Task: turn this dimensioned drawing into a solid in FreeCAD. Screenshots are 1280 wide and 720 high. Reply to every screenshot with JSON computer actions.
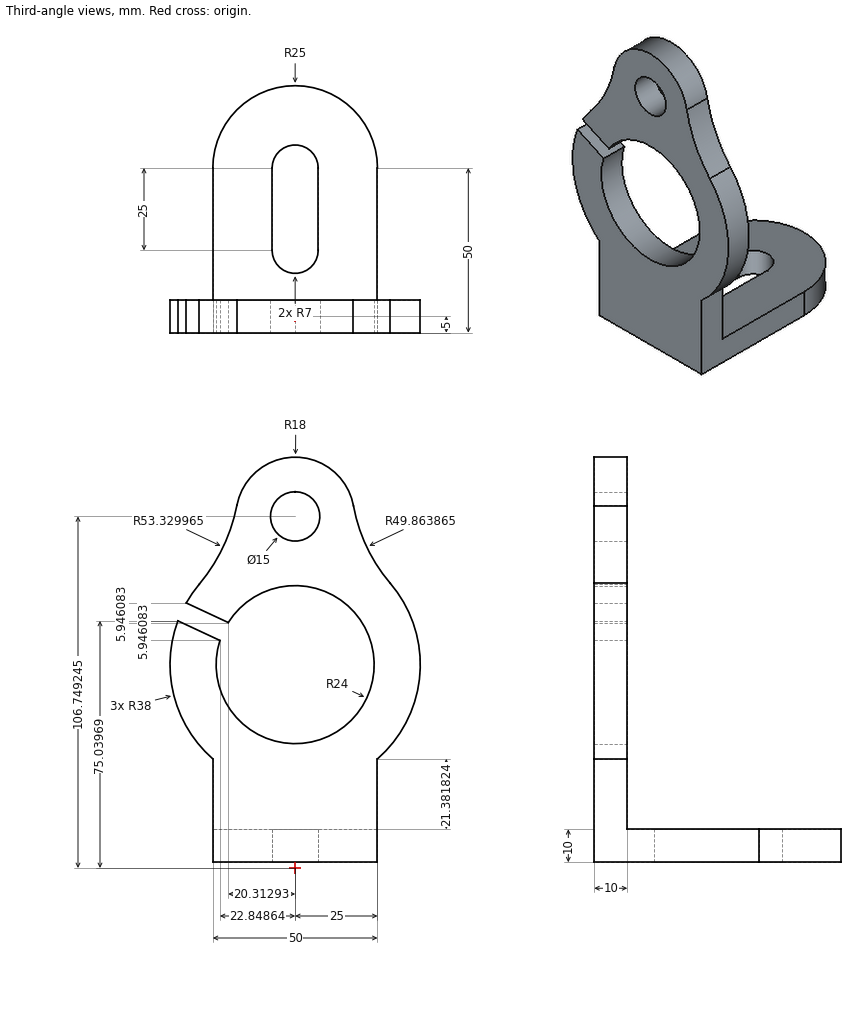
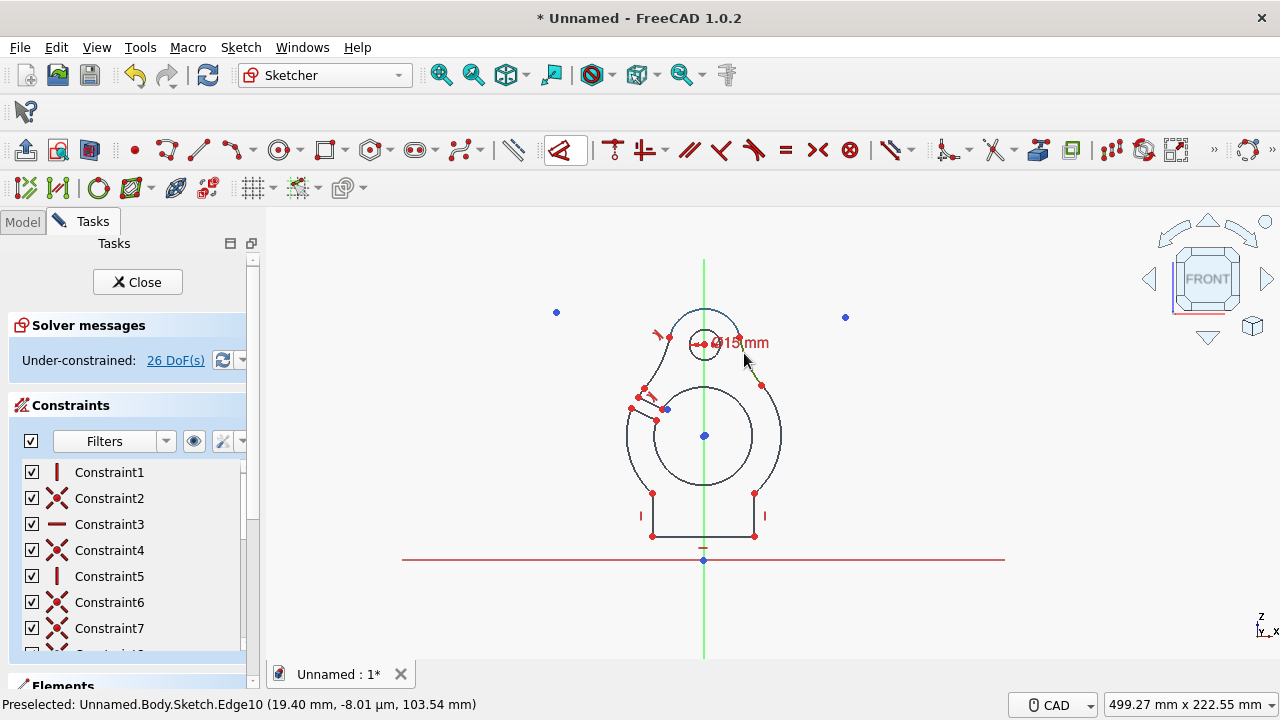
{"action": "left_click", "coordinate": [754, 150]}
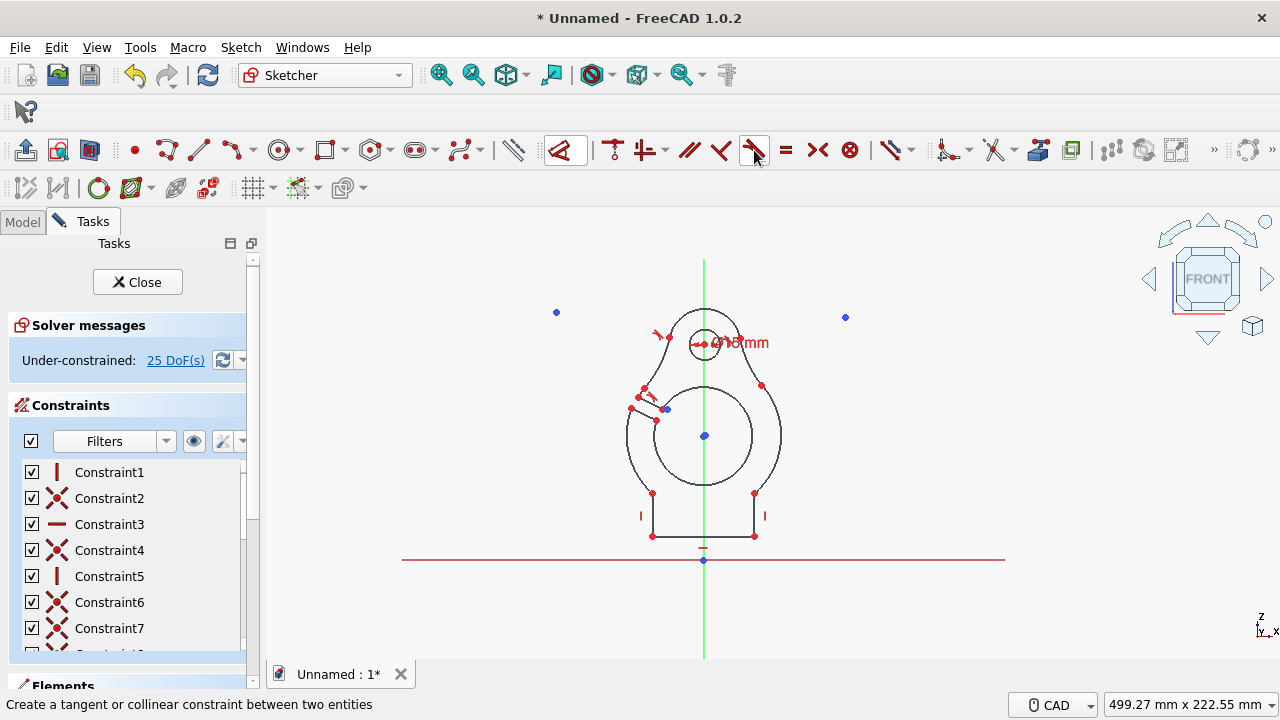
{"action": "left_click", "coordinate": [744, 353]}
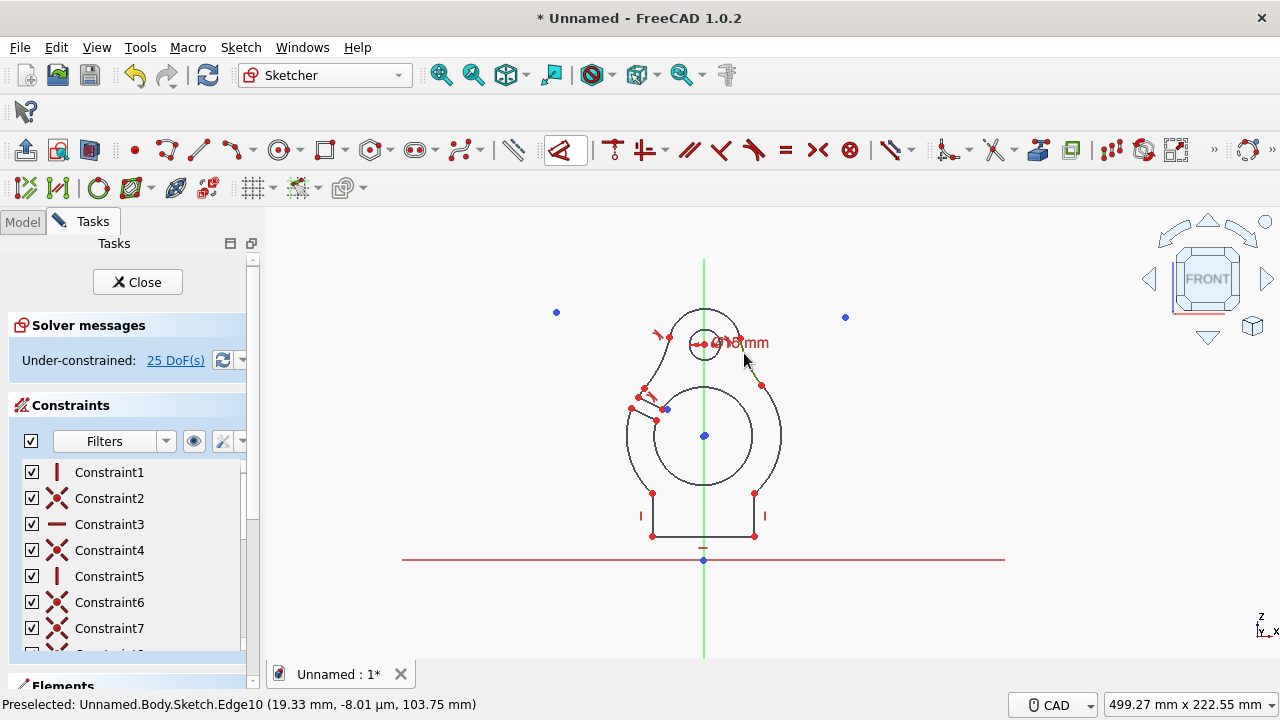
{"action": "left_click", "coordinate": [775, 465]}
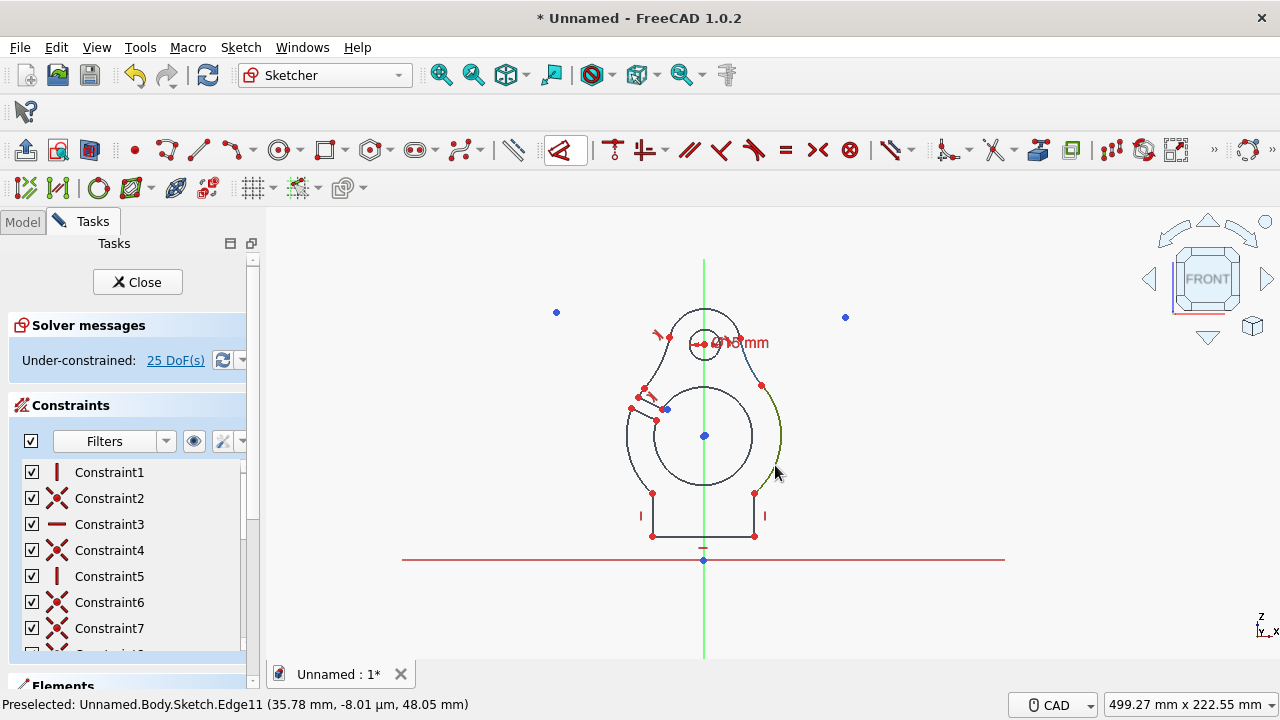
{"action": "key", "text": "t"}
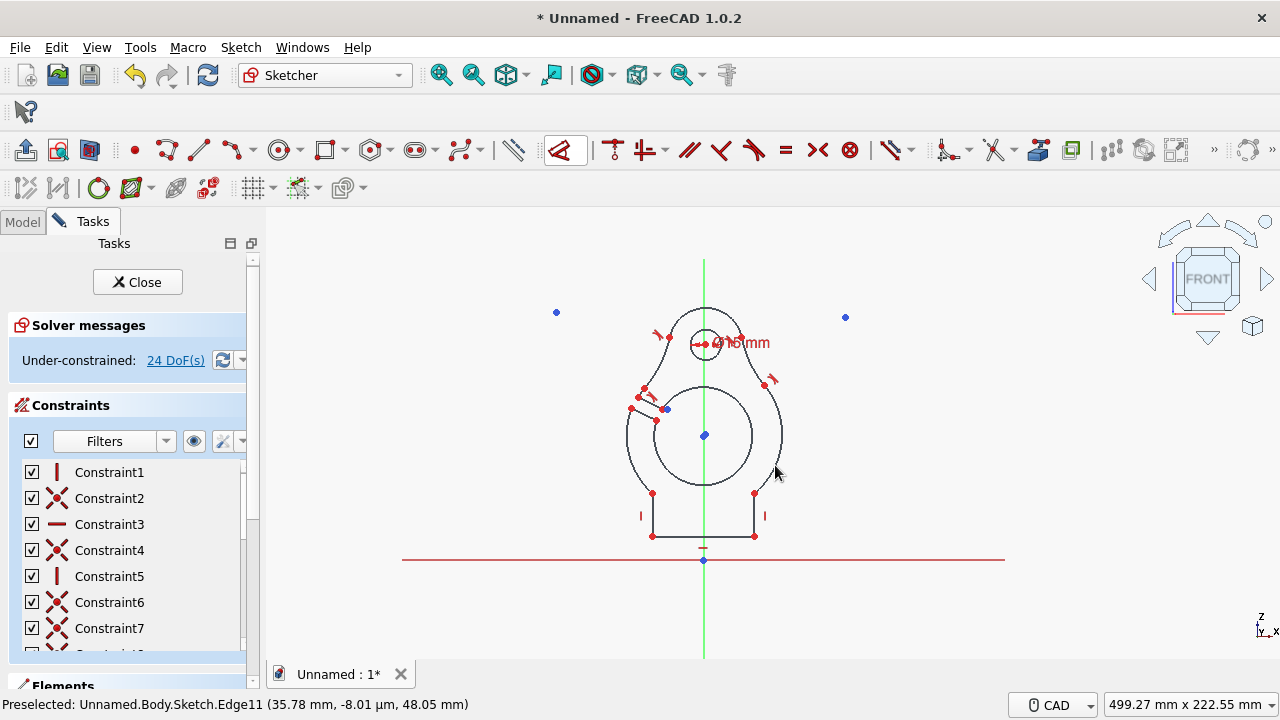
{"action": "left_click", "coordinate": [739, 403]}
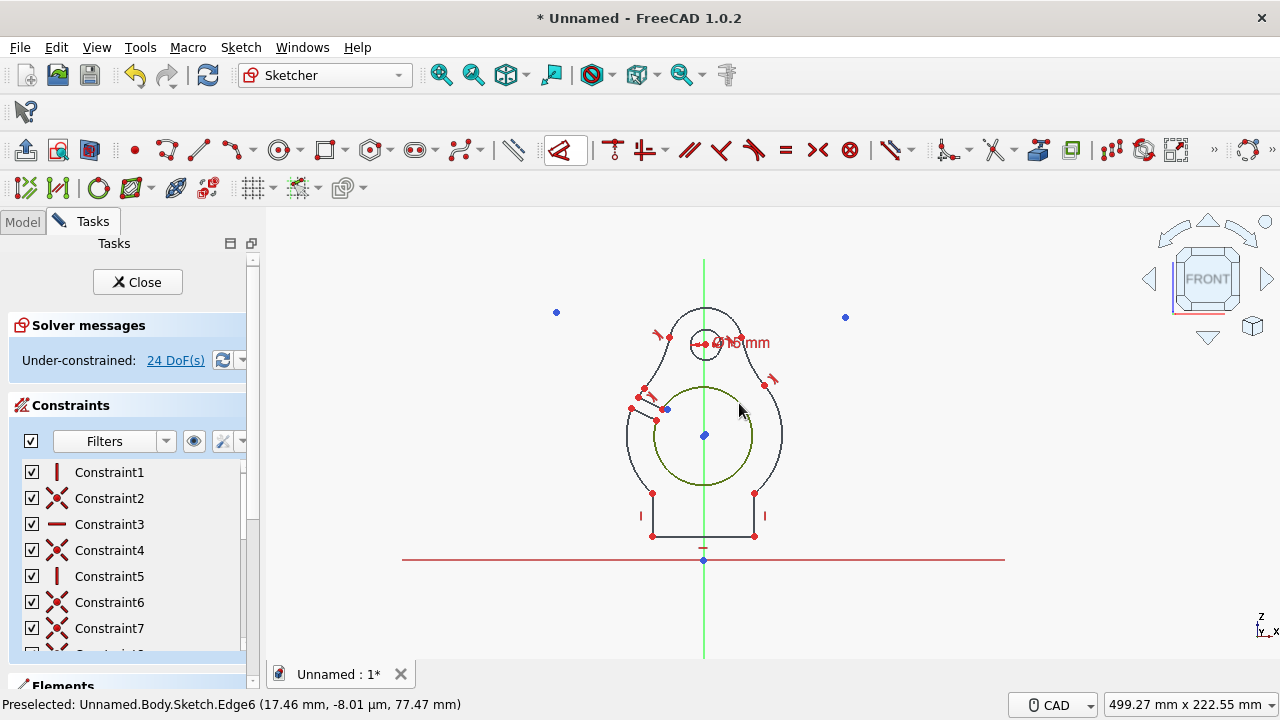
{"action": "scroll", "coordinate": [641, 393], "scroll_direction": "up", "scroll_amount": 6}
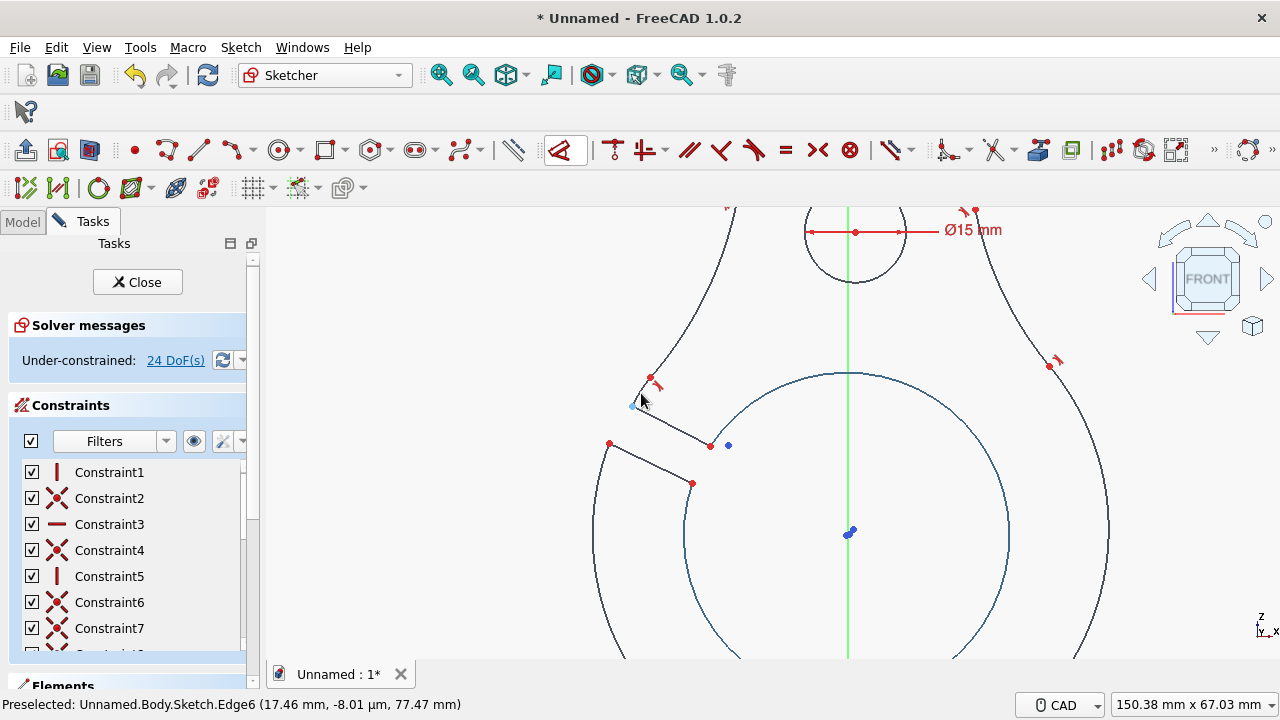
{"action": "left_click", "coordinate": [640, 391]}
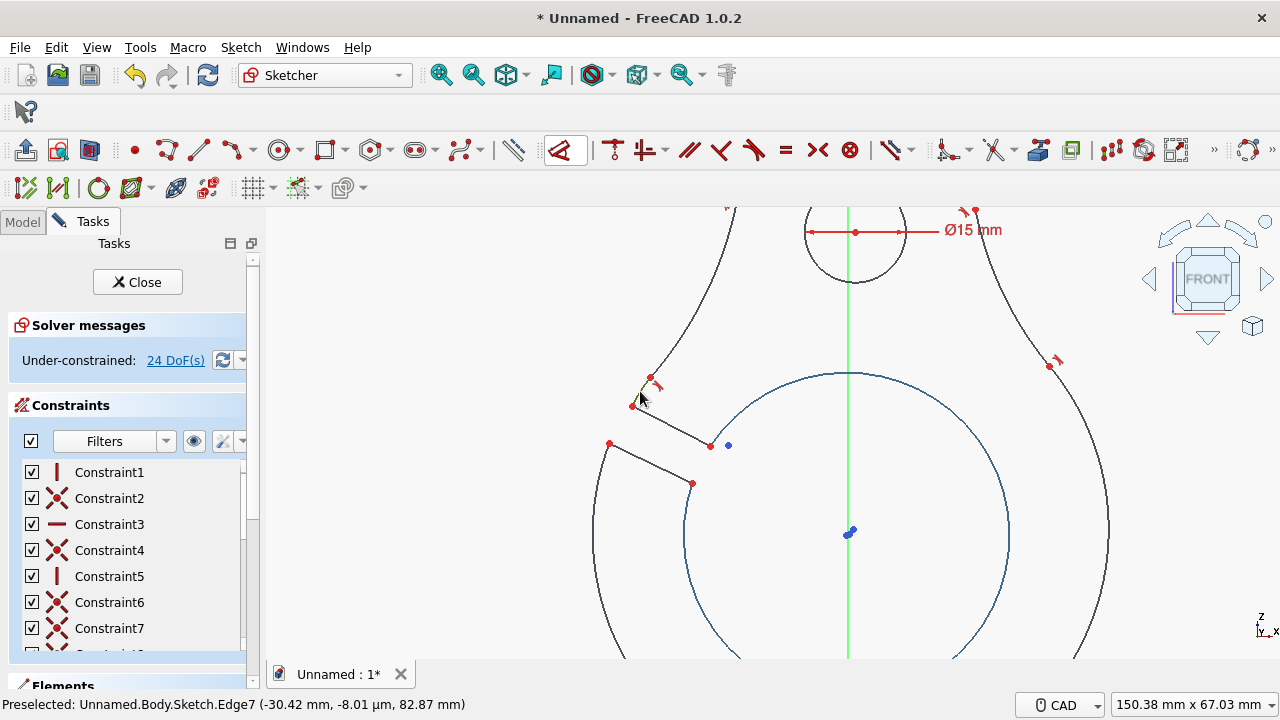
{"action": "left_click", "coordinate": [614, 150]}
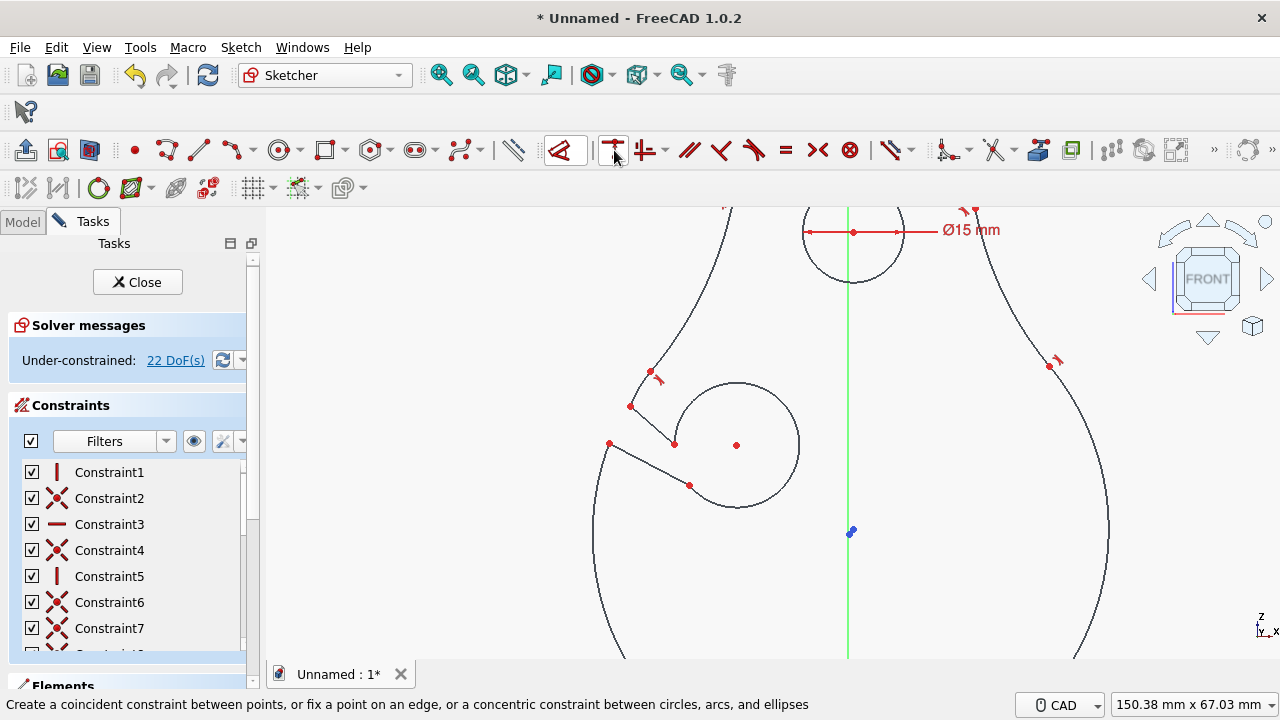
{"action": "left_click", "coordinate": [782, 489]}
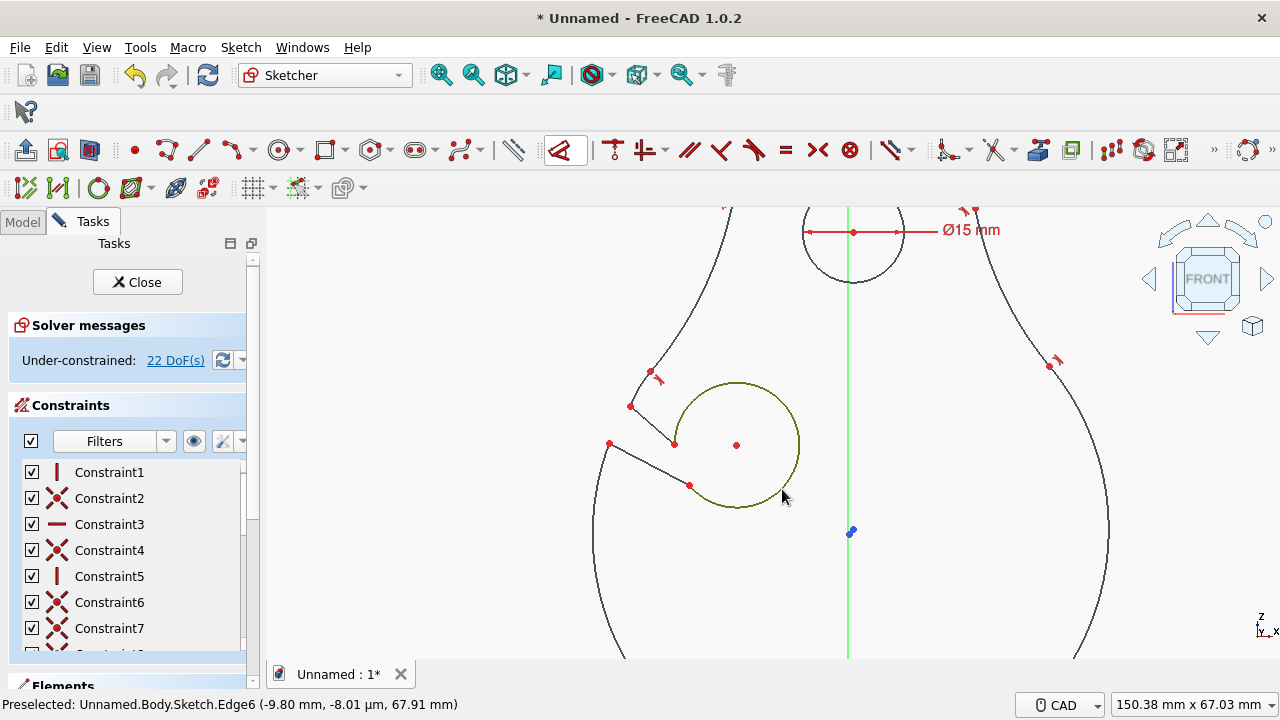
{"action": "left_click", "coordinate": [1103, 474]}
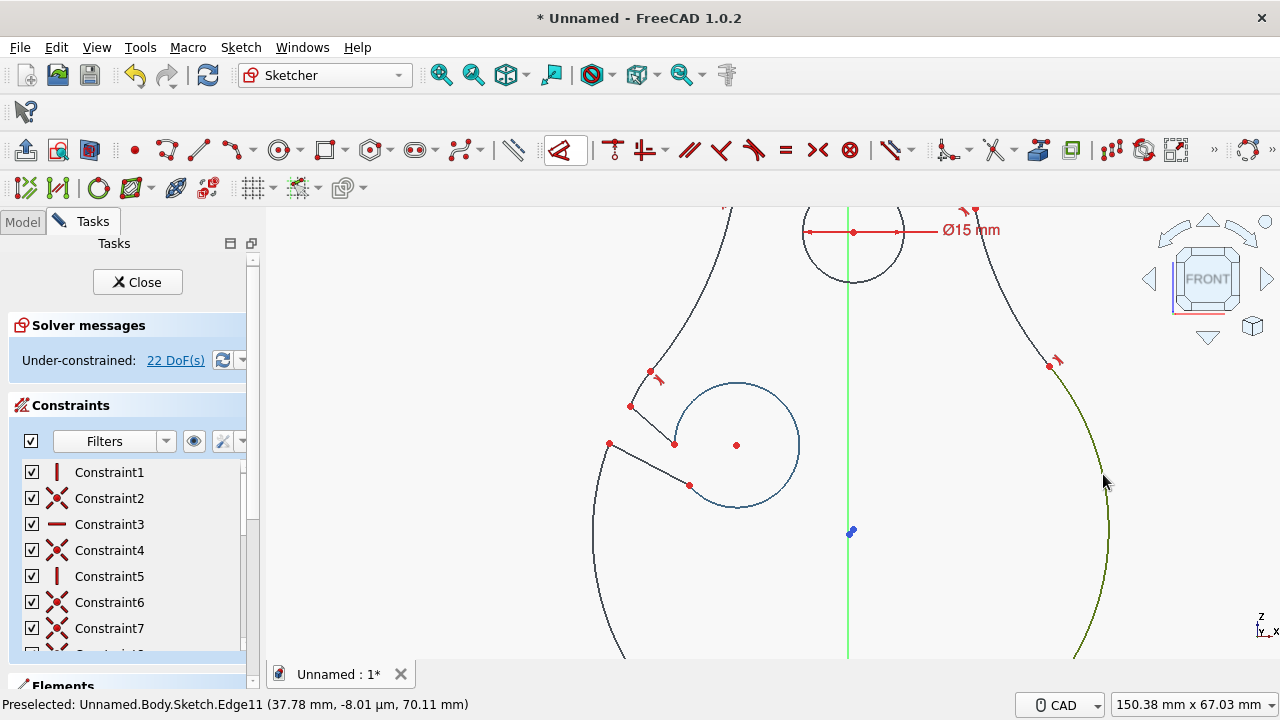
{"action": "left_click", "coordinate": [614, 150]}